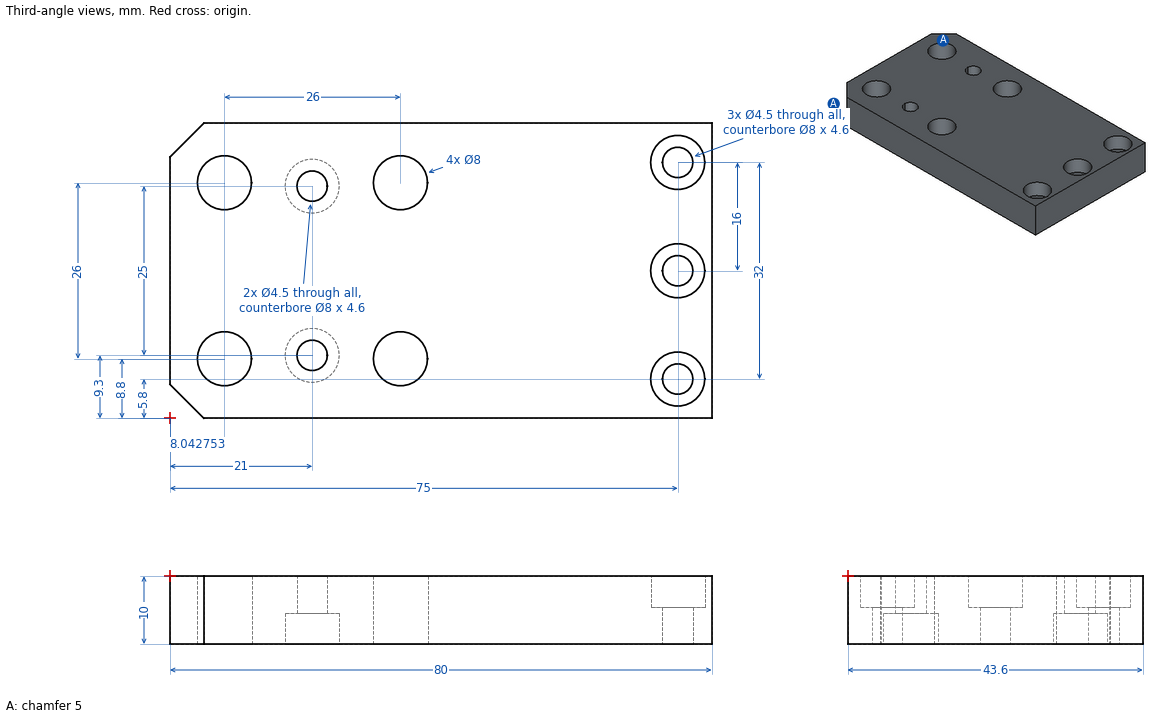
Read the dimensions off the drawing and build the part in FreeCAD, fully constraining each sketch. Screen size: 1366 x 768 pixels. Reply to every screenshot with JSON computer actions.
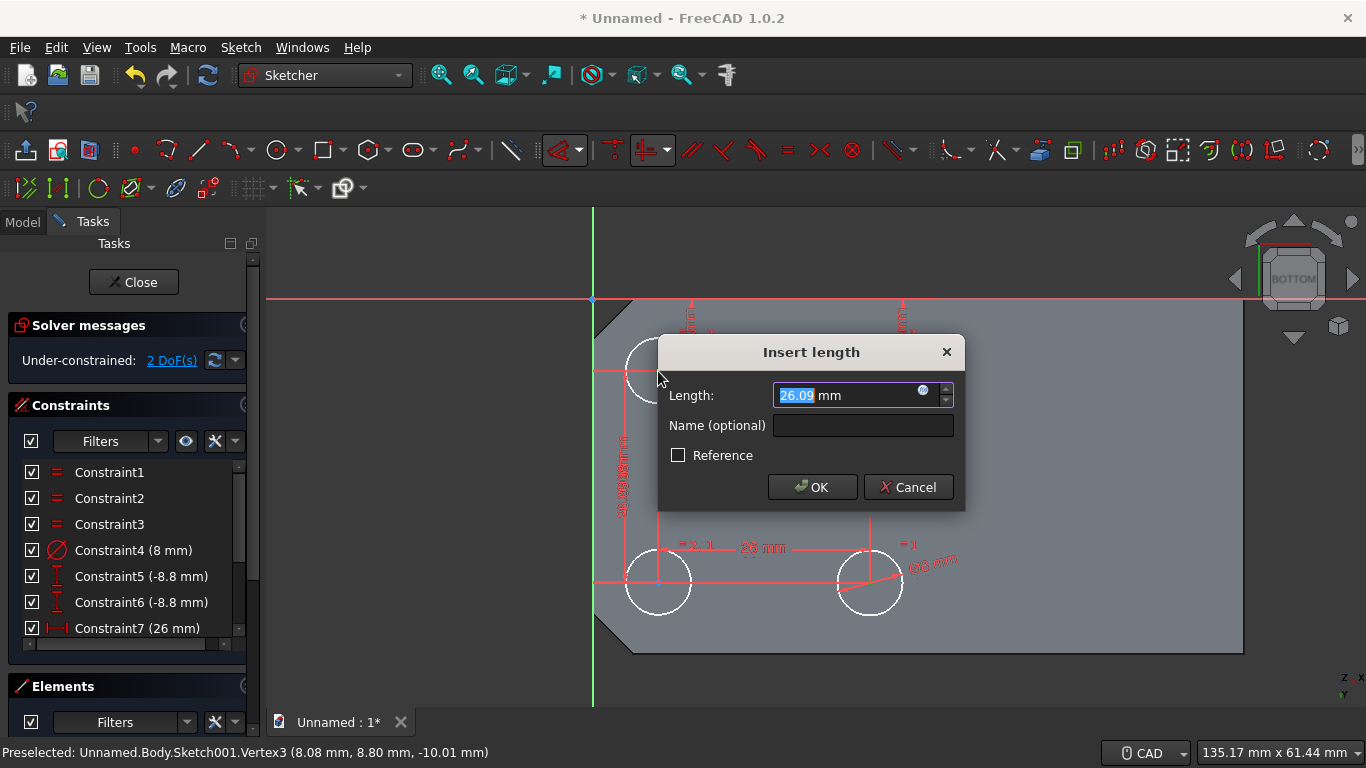
{"action": "type", "text": "26"}
{"action": "key", "text": "Return"}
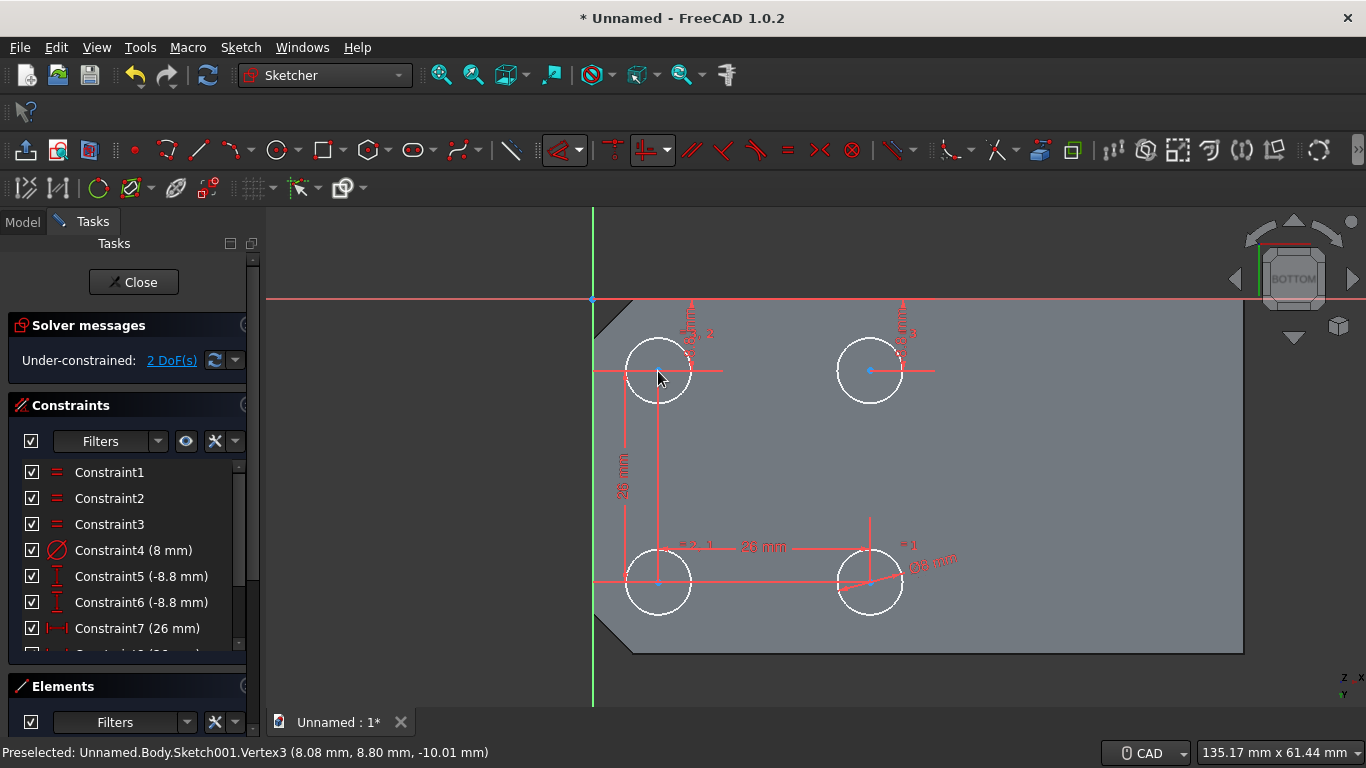
{"action": "left_click", "coordinate": [658, 371]}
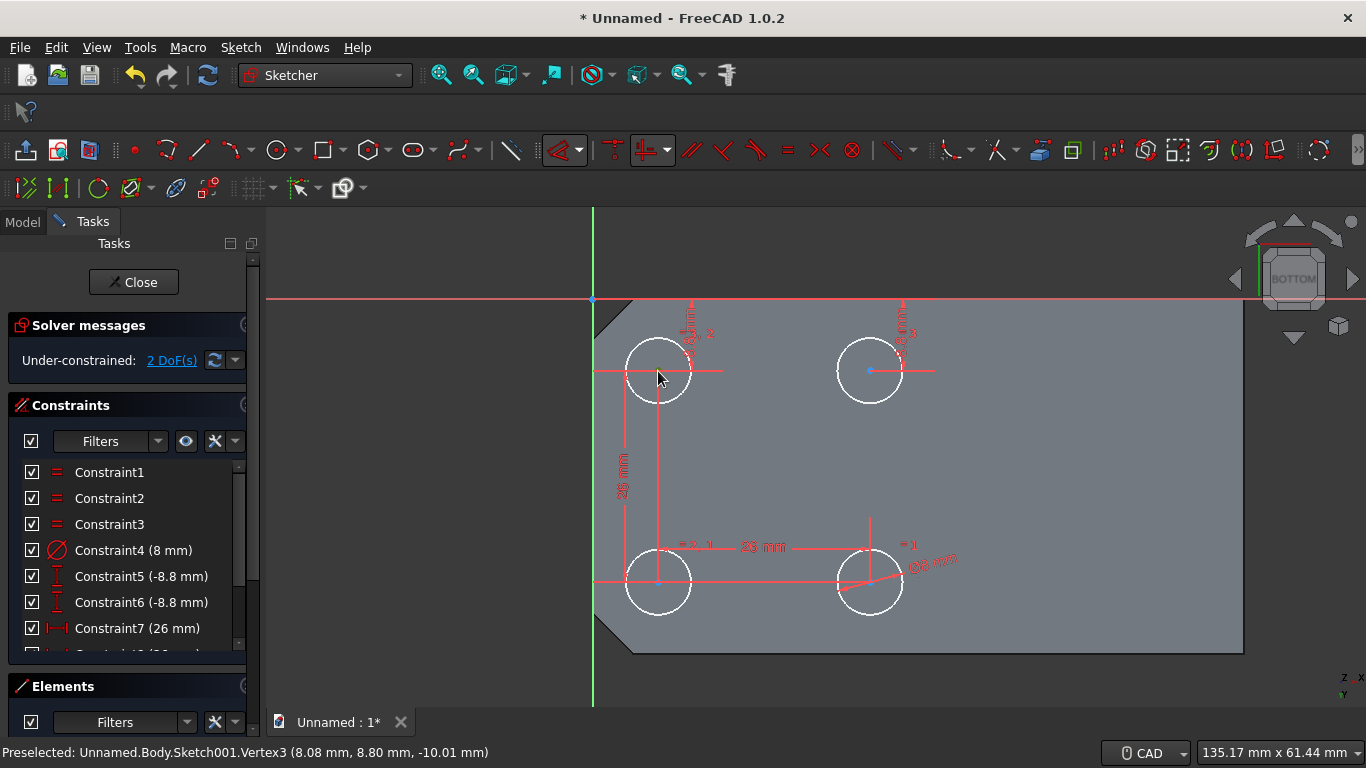
{"action": "left_click", "coordinate": [870, 371]}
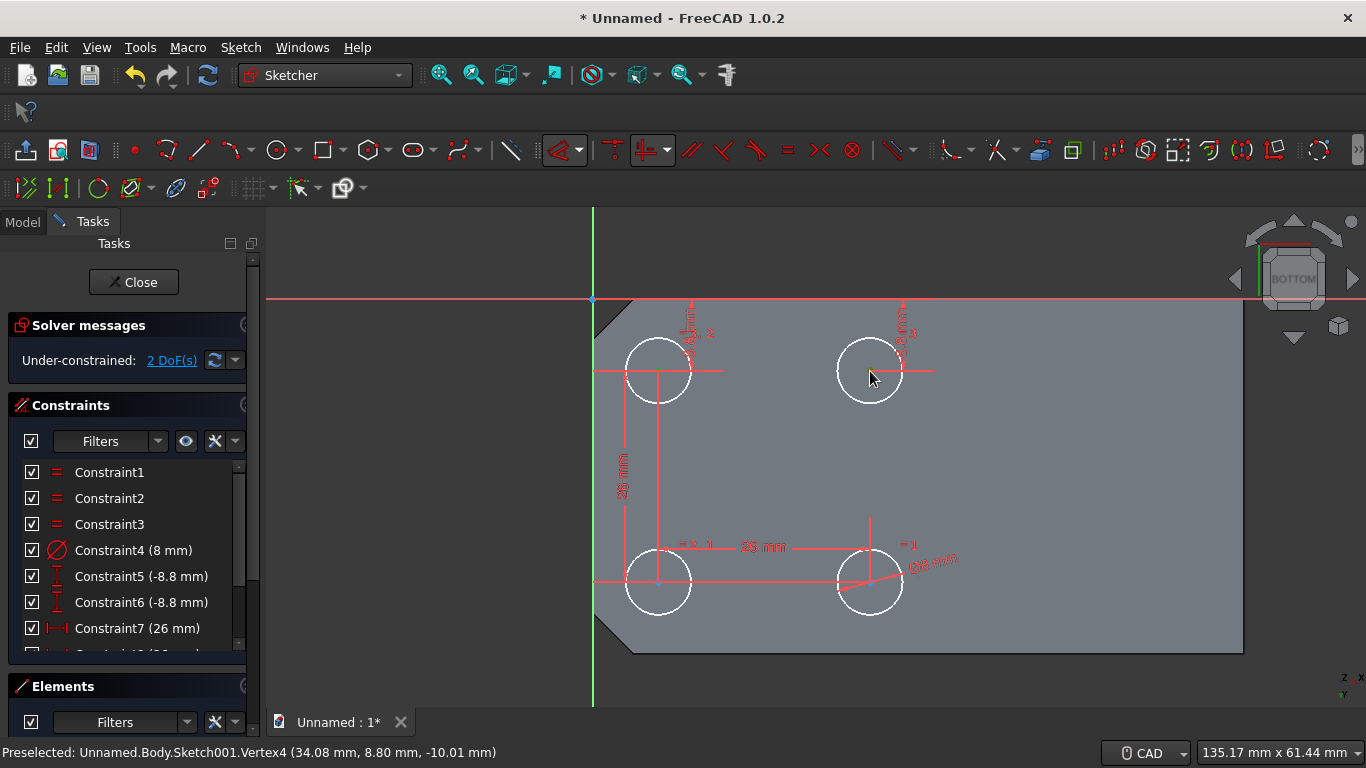
{"action": "left_click", "coordinate": [582, 150]}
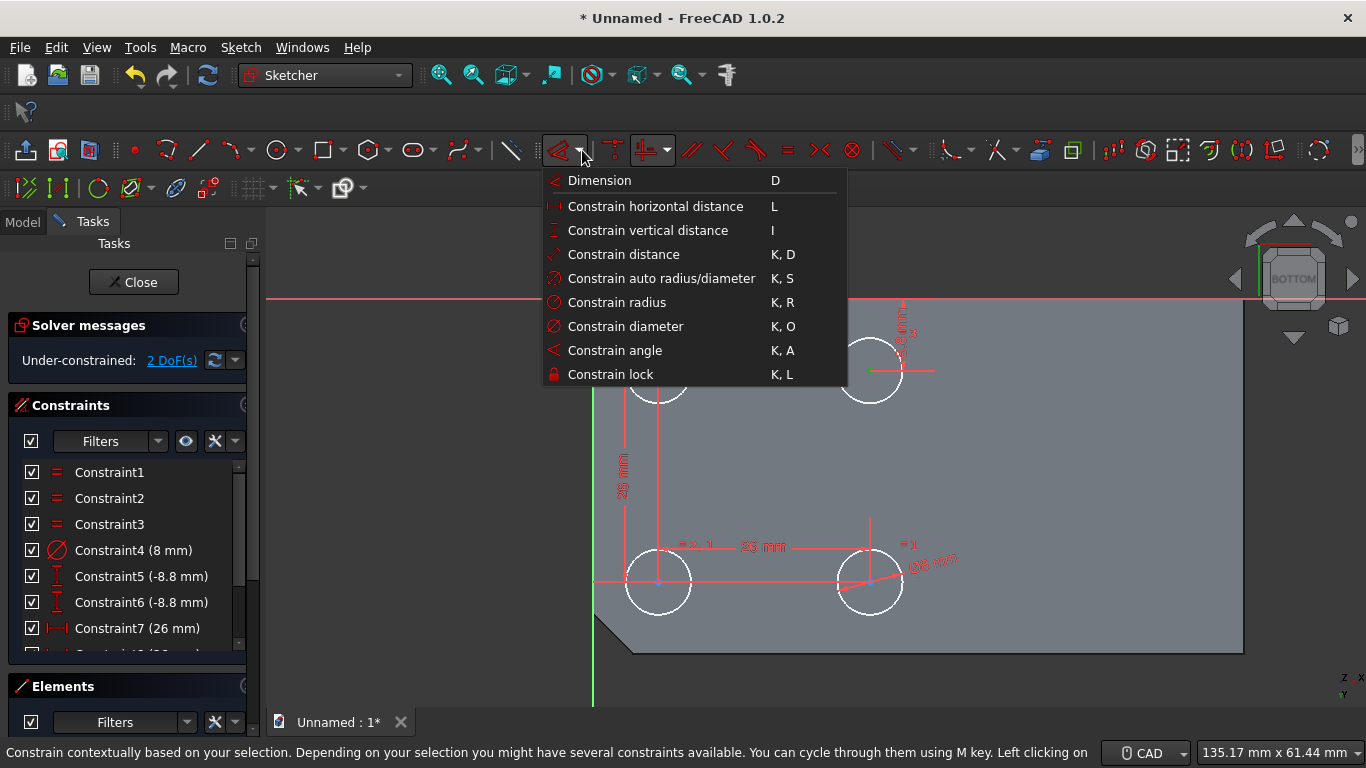
{"action": "left_click", "coordinate": [695, 206]}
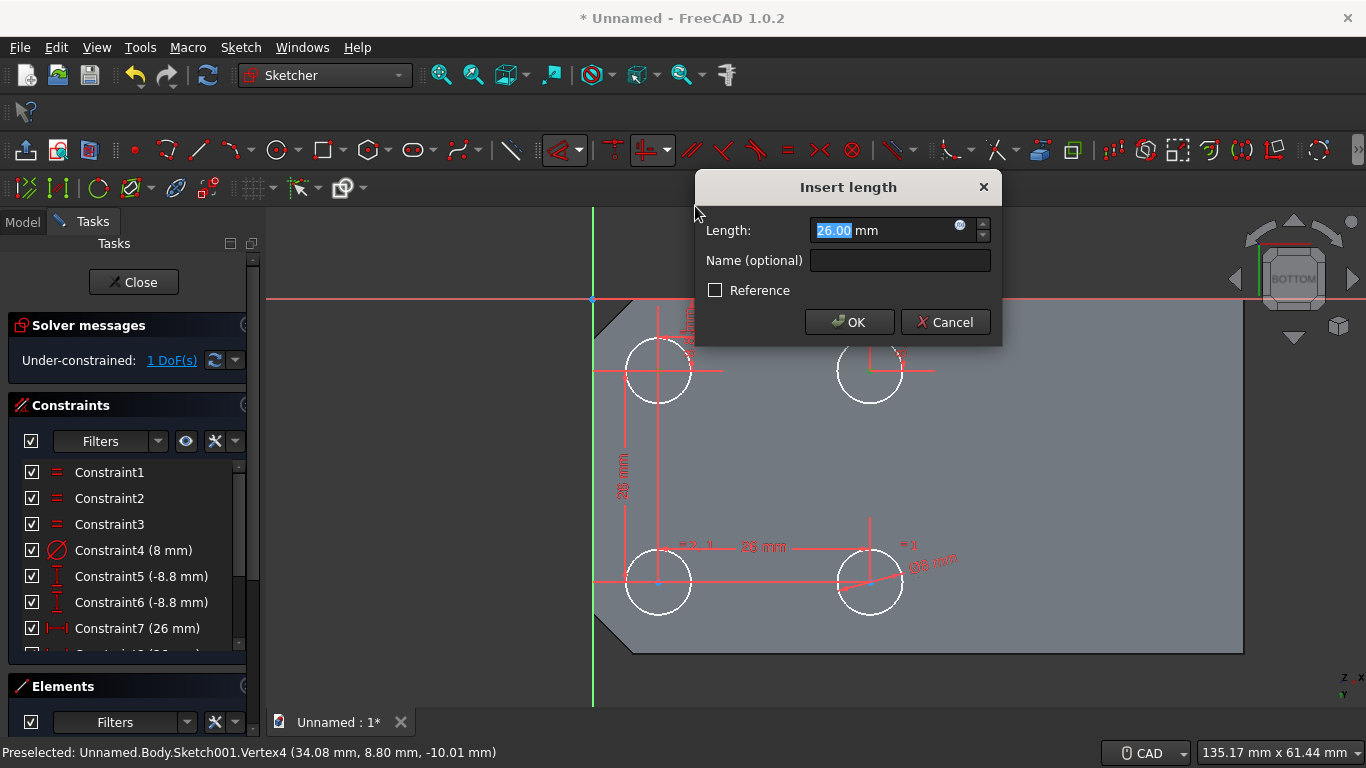
{"action": "type", "text": "26"}
{"action": "key", "text": "Return"}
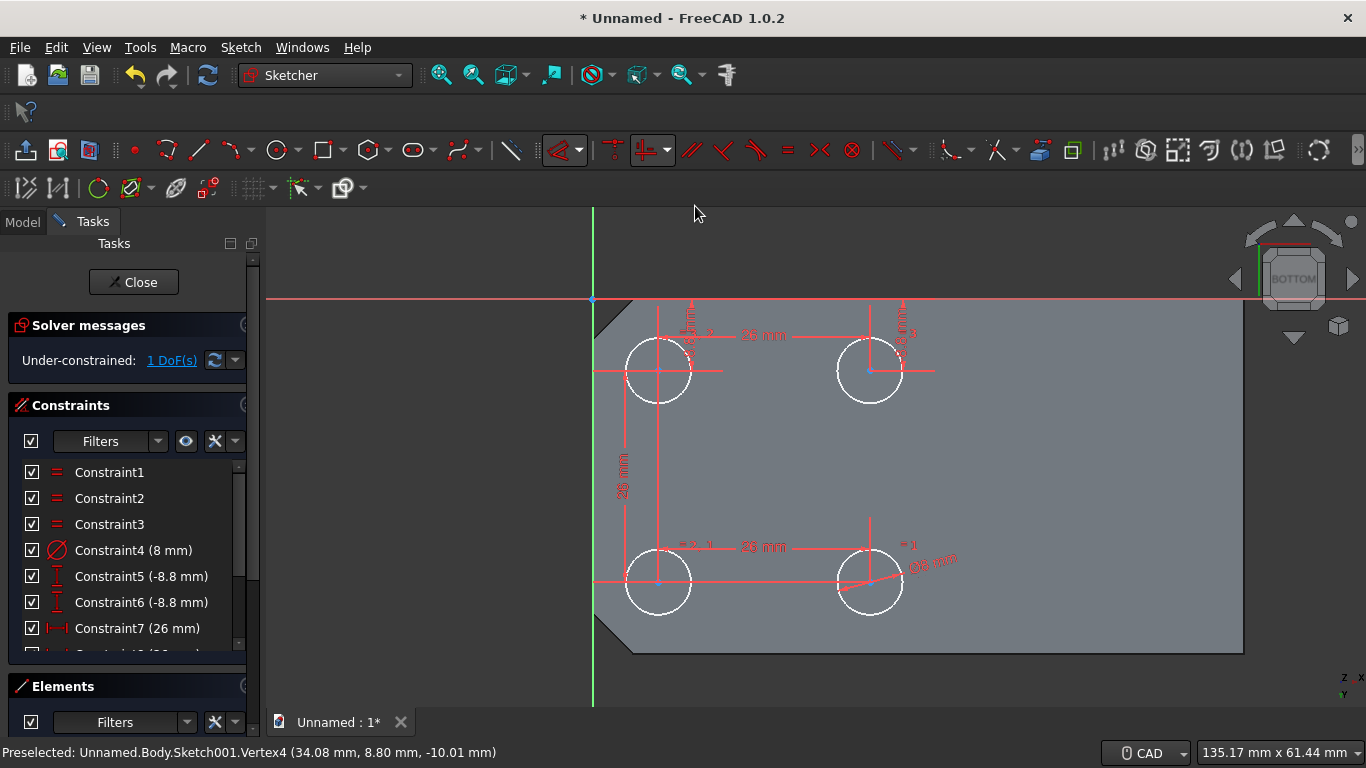
{"action": "left_click", "coordinate": [658, 582]}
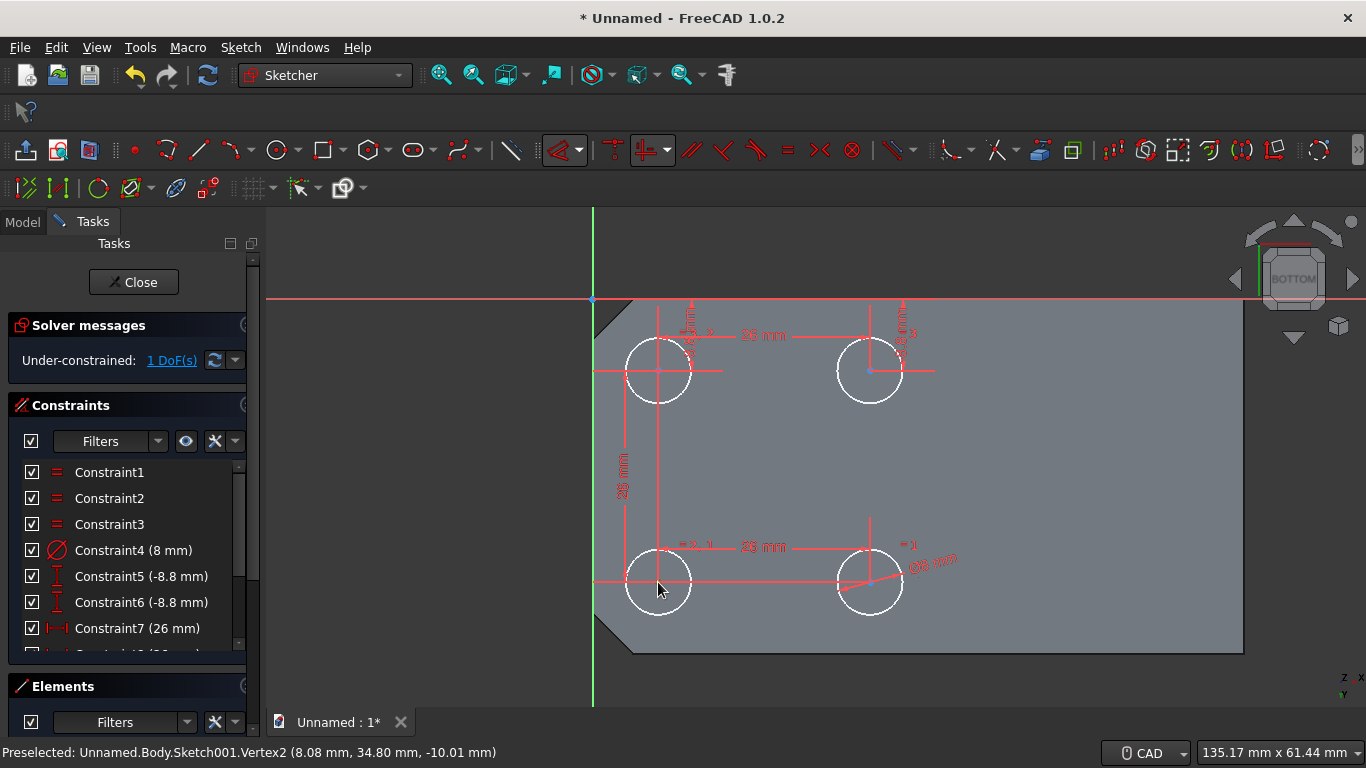
{"action": "key", "text": "l"}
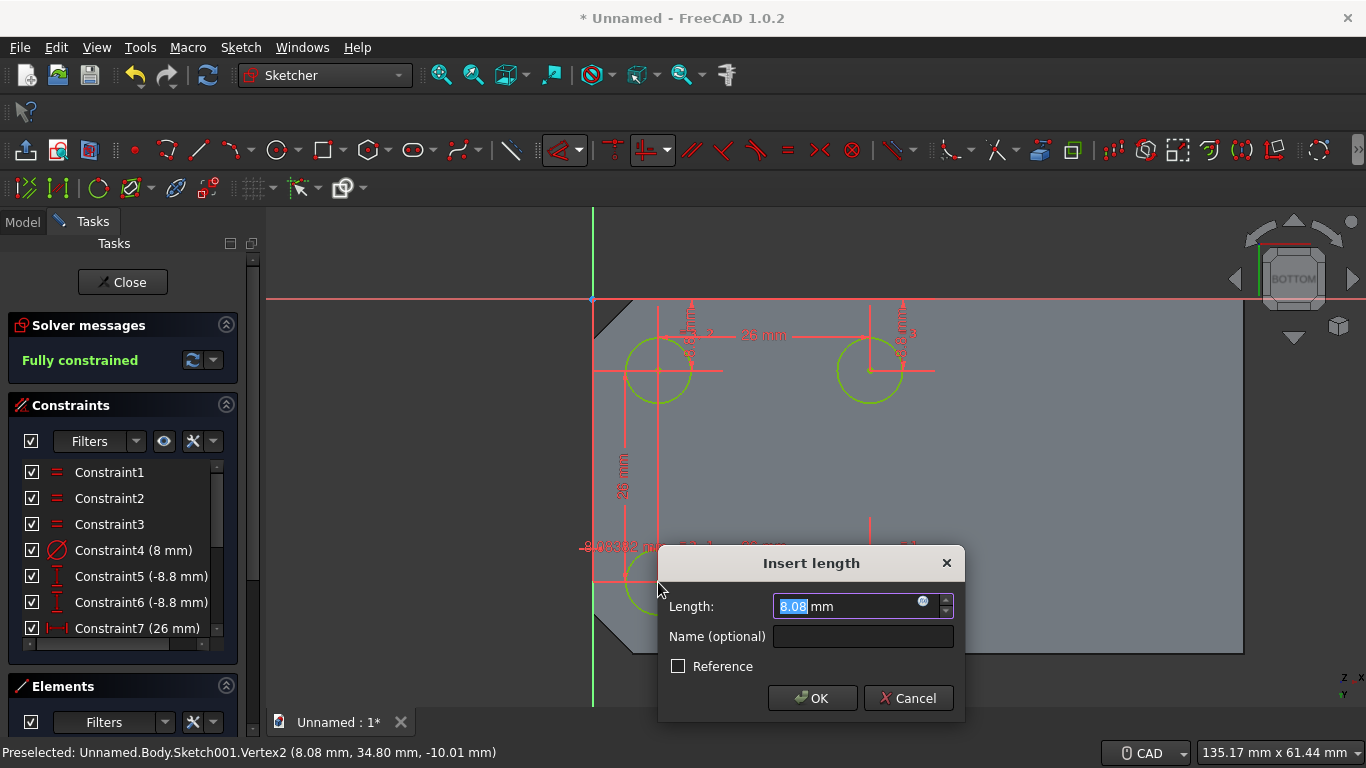
{"action": "type", "text": "8.042753"}
{"action": "key", "text": "Return"}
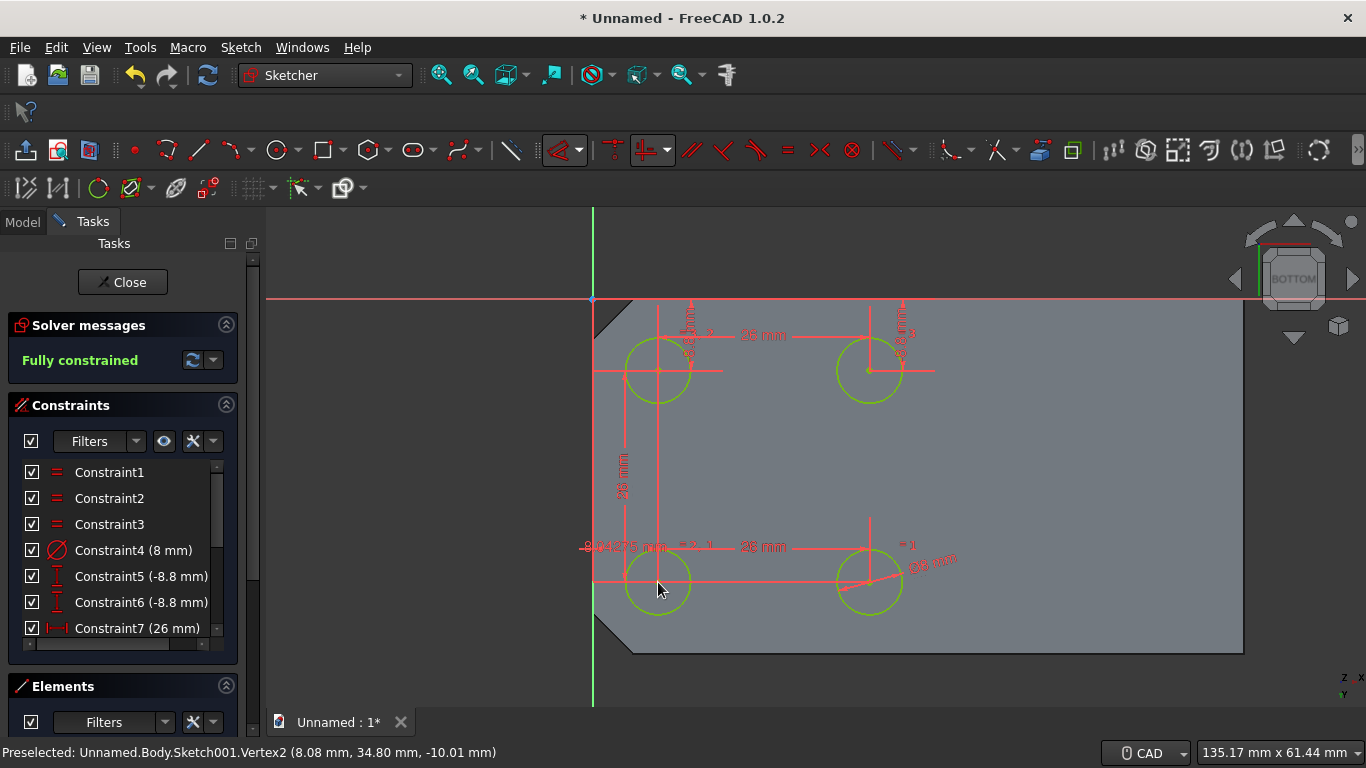
{"action": "left_click", "coordinate": [123, 282]}